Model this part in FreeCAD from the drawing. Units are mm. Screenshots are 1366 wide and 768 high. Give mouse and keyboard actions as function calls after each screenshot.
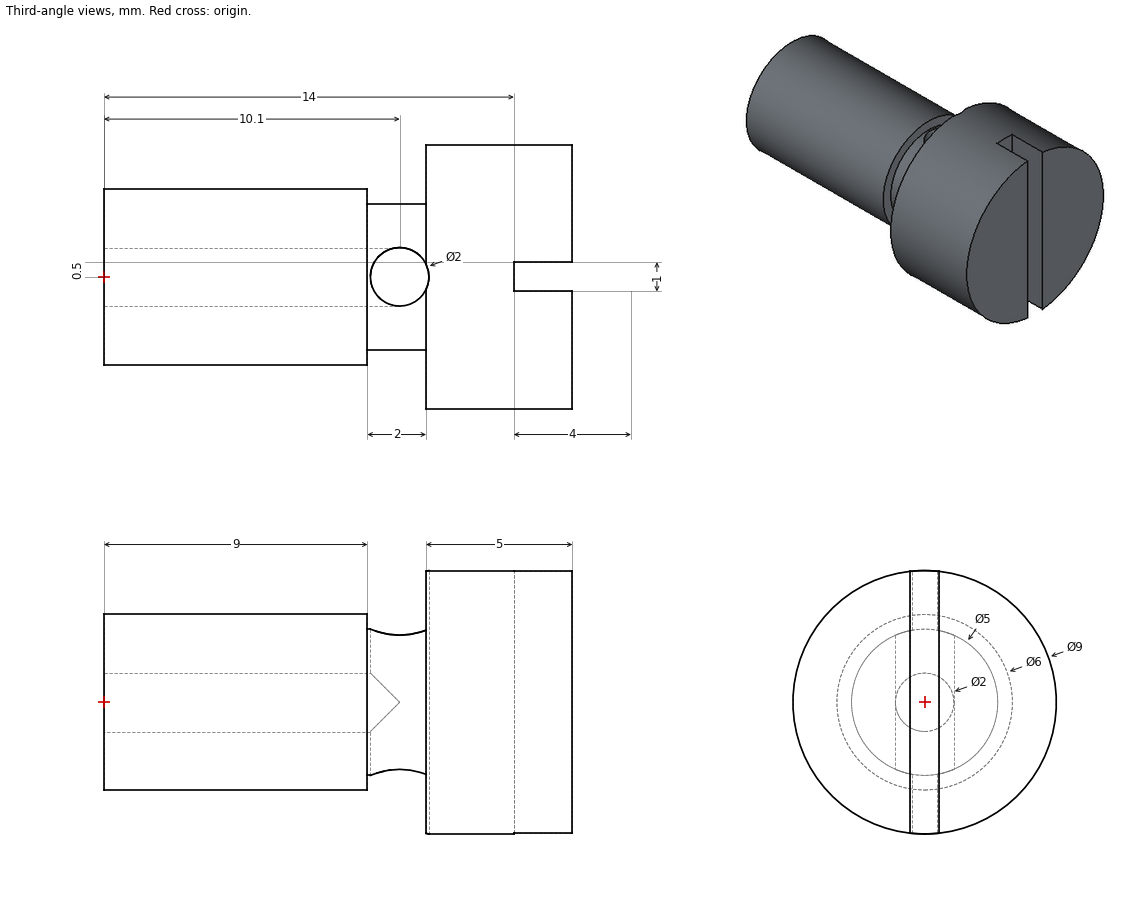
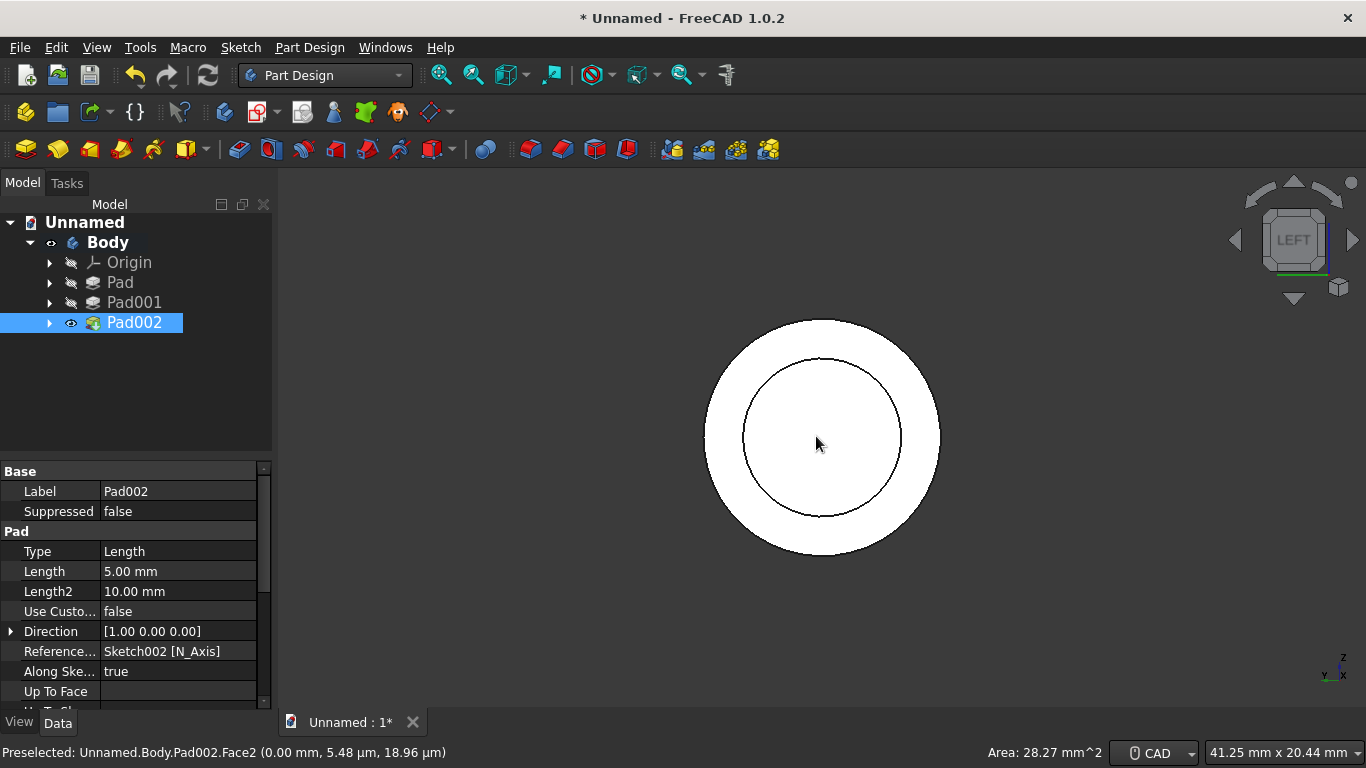
click(258, 112)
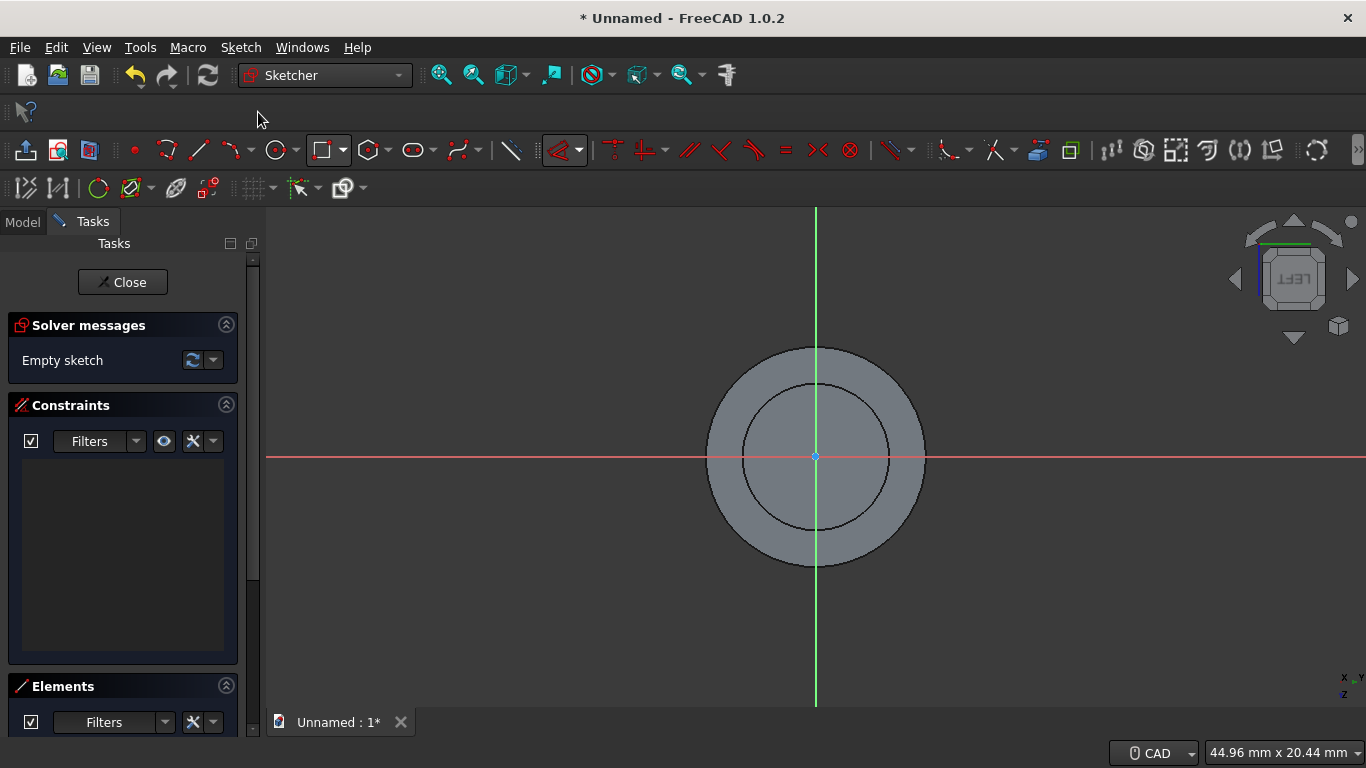
scroll(829, 457, up, 9)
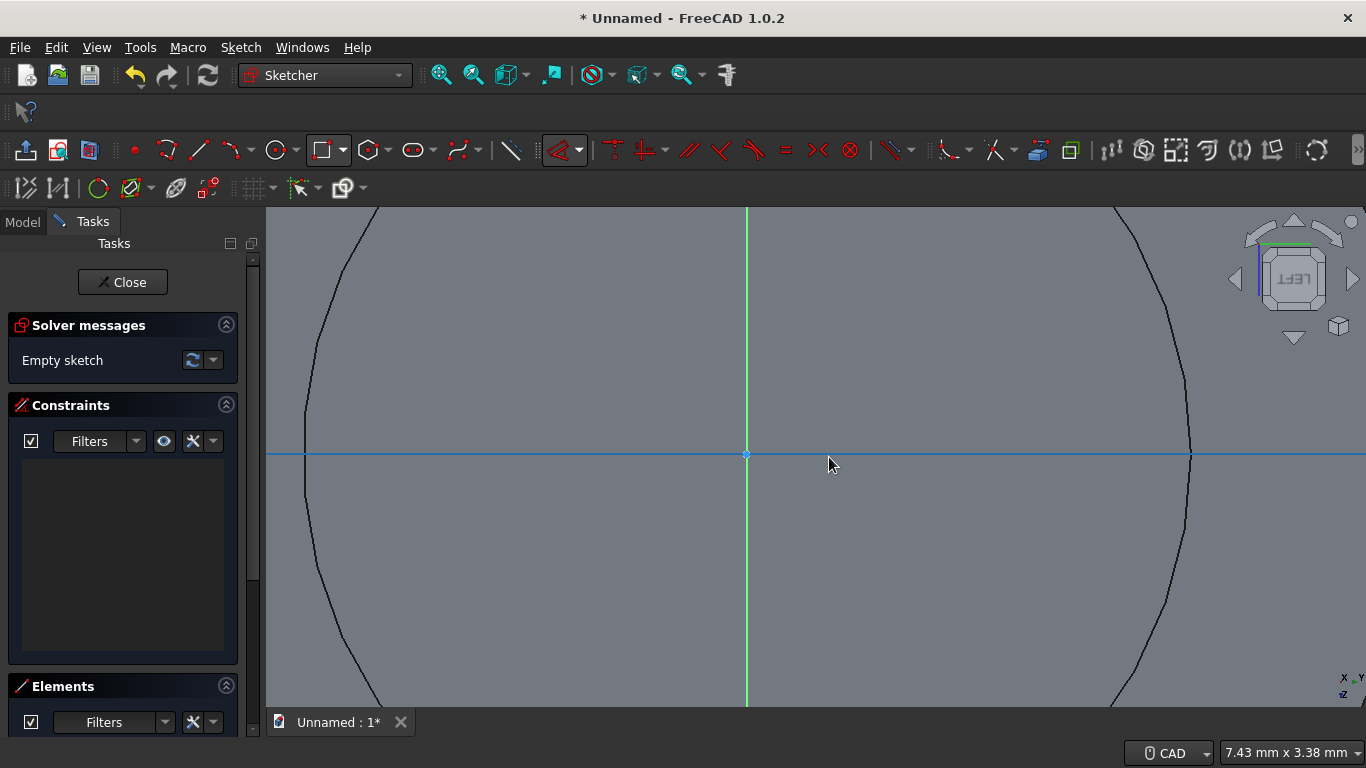
click(276, 150)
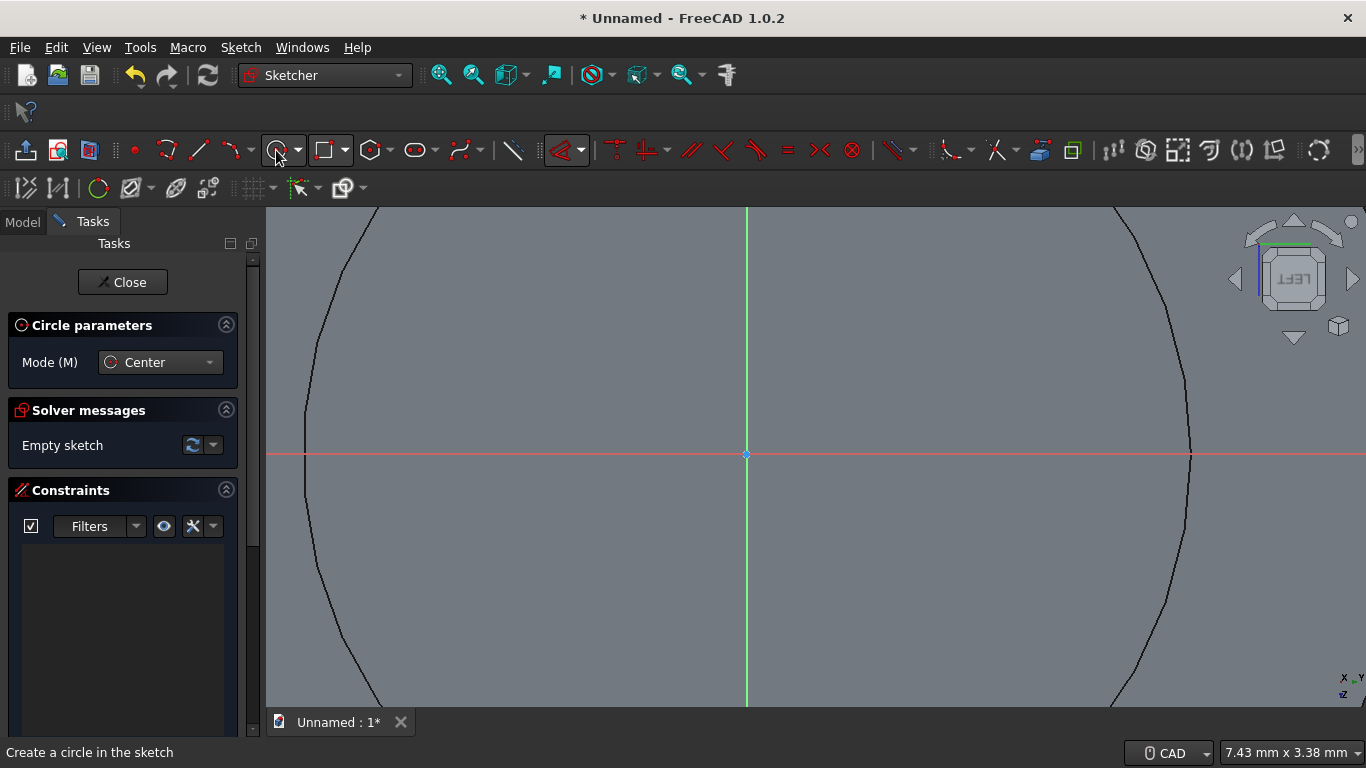
click(747, 454)
click(852, 350)
key(Escape)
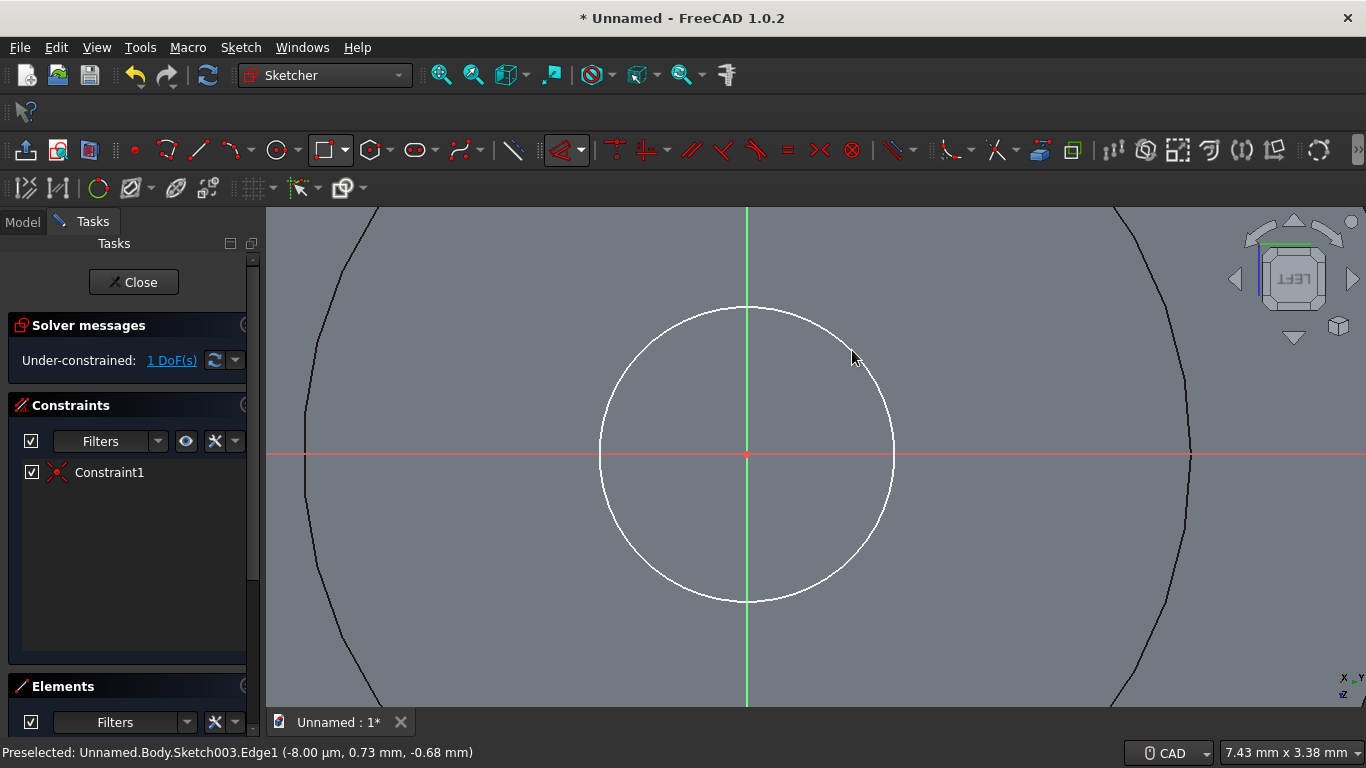
click(851, 350)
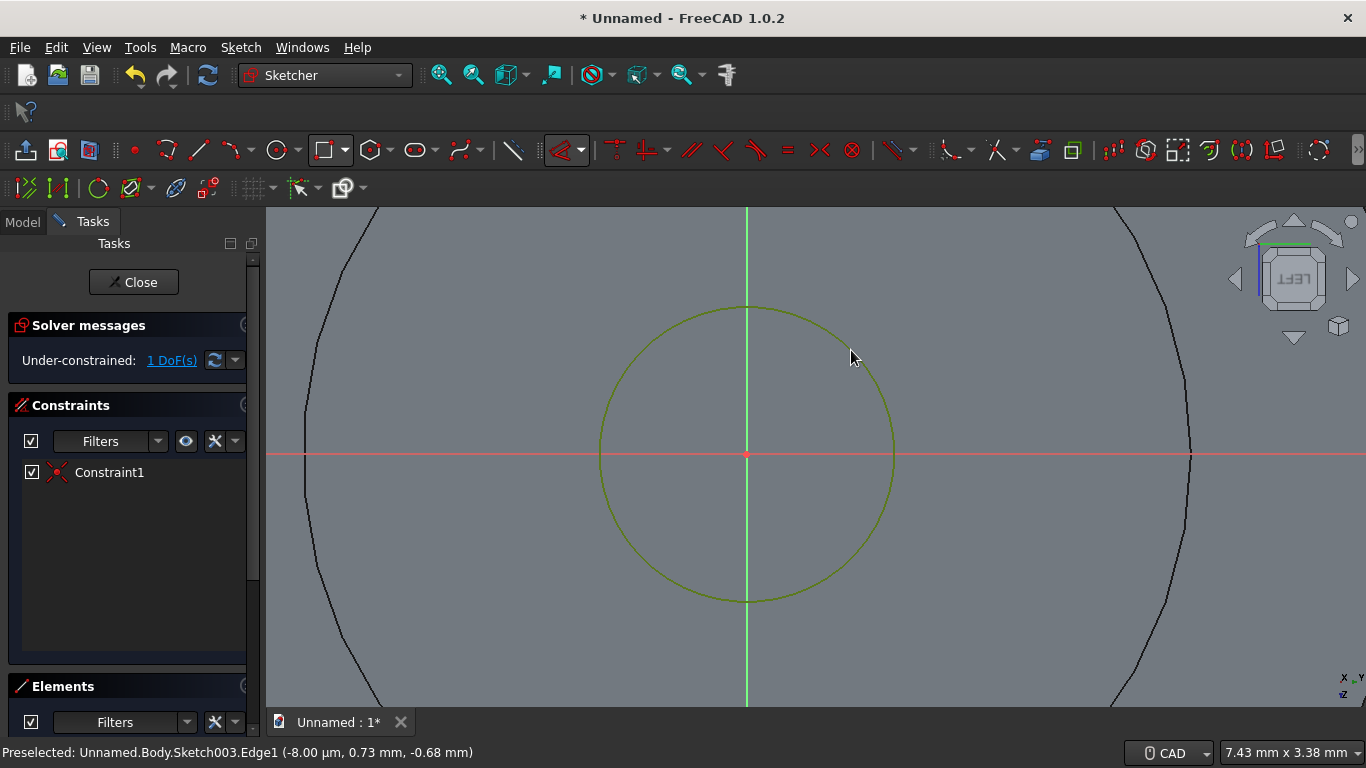
click(584, 150)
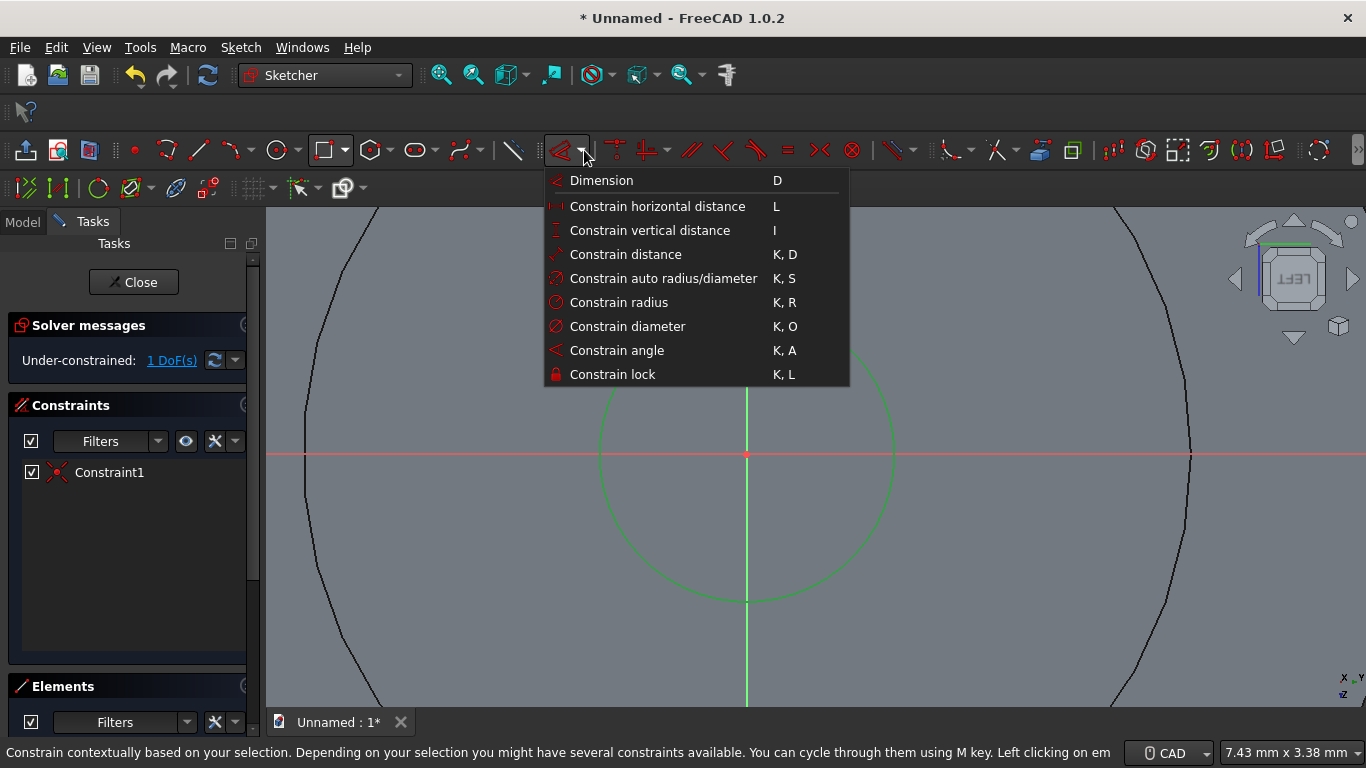
click(697, 326)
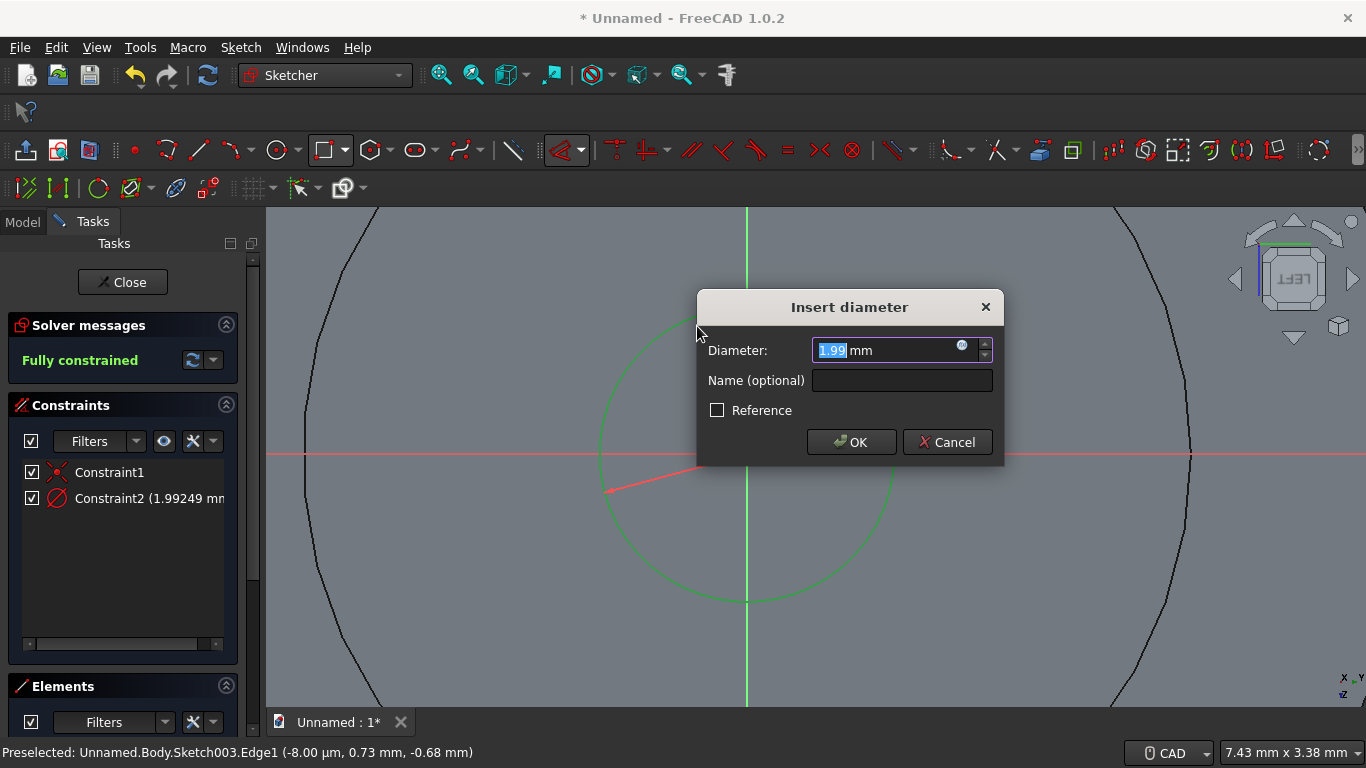
text(2)
key(Return)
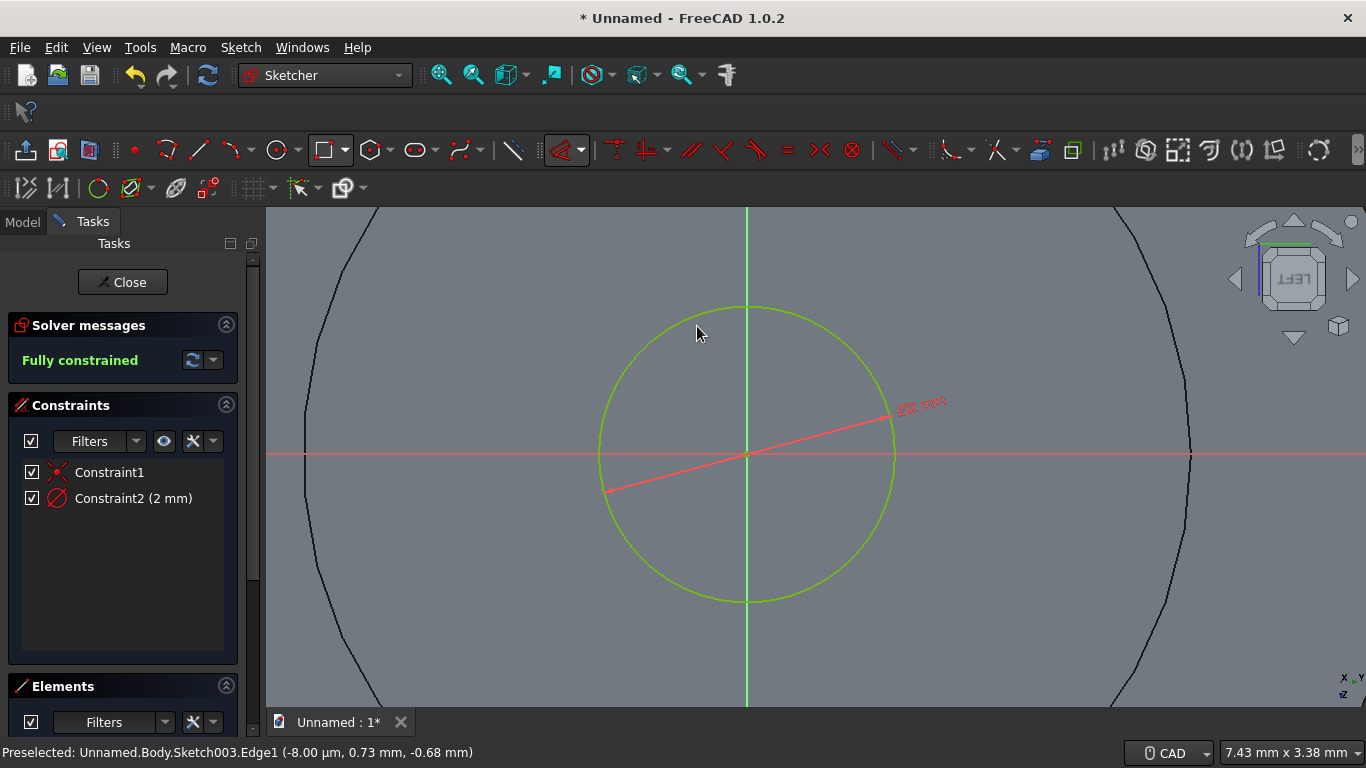
click(123, 282)